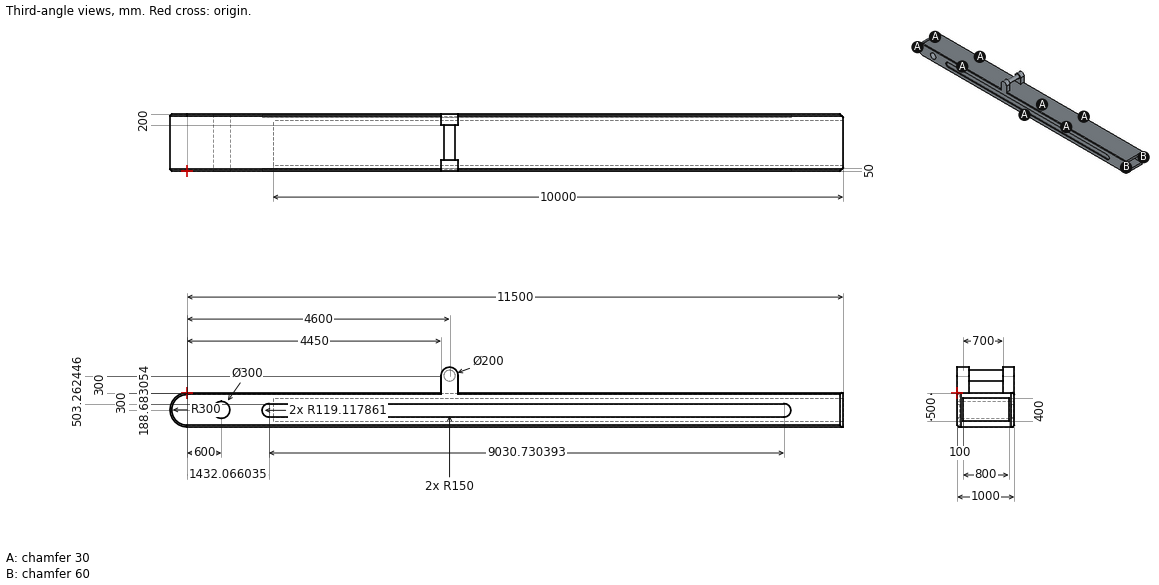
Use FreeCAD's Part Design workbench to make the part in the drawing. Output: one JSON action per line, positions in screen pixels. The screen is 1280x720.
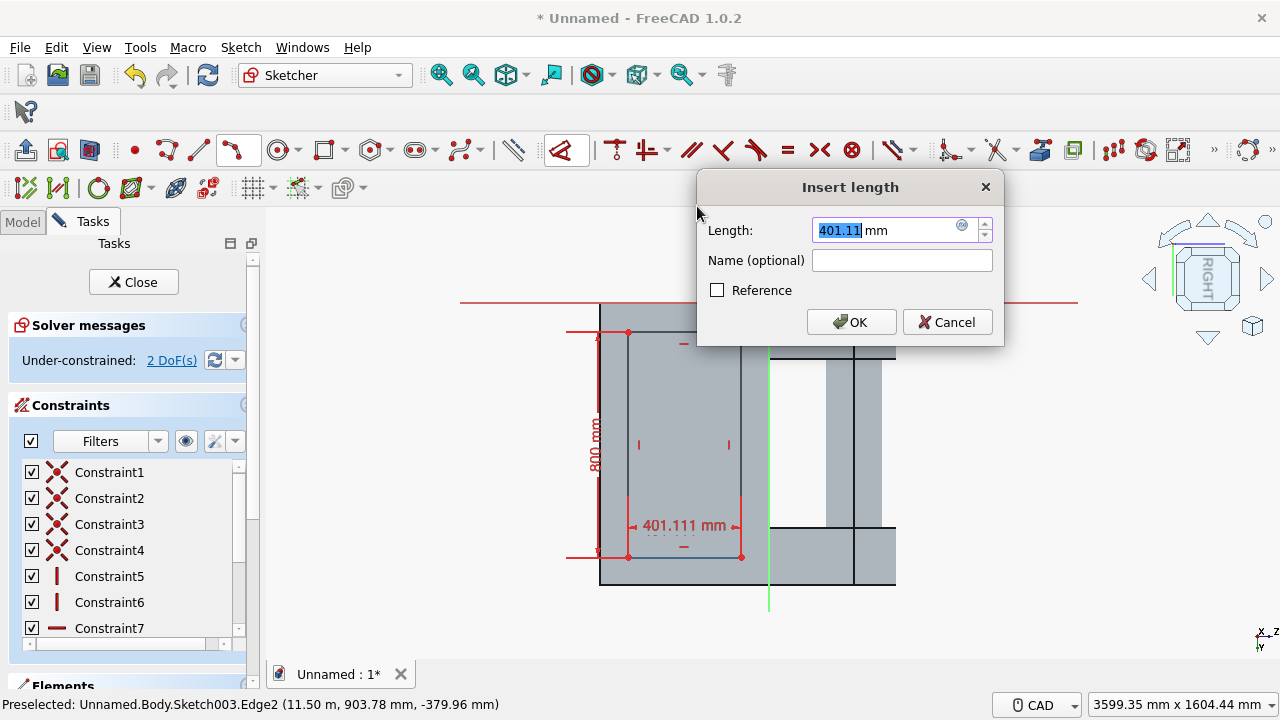
{"action": "type", "text": "400"}
{"action": "key", "text": "Return"}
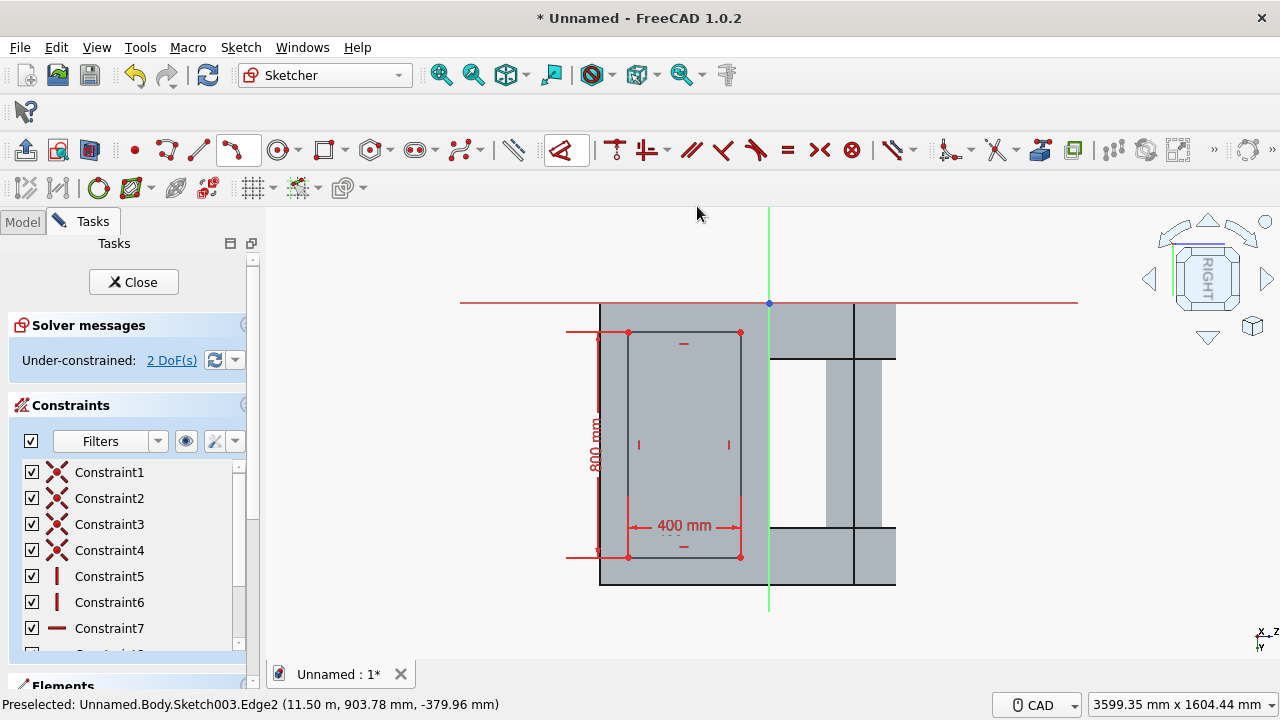
{"action": "left_click", "coordinate": [628, 332]}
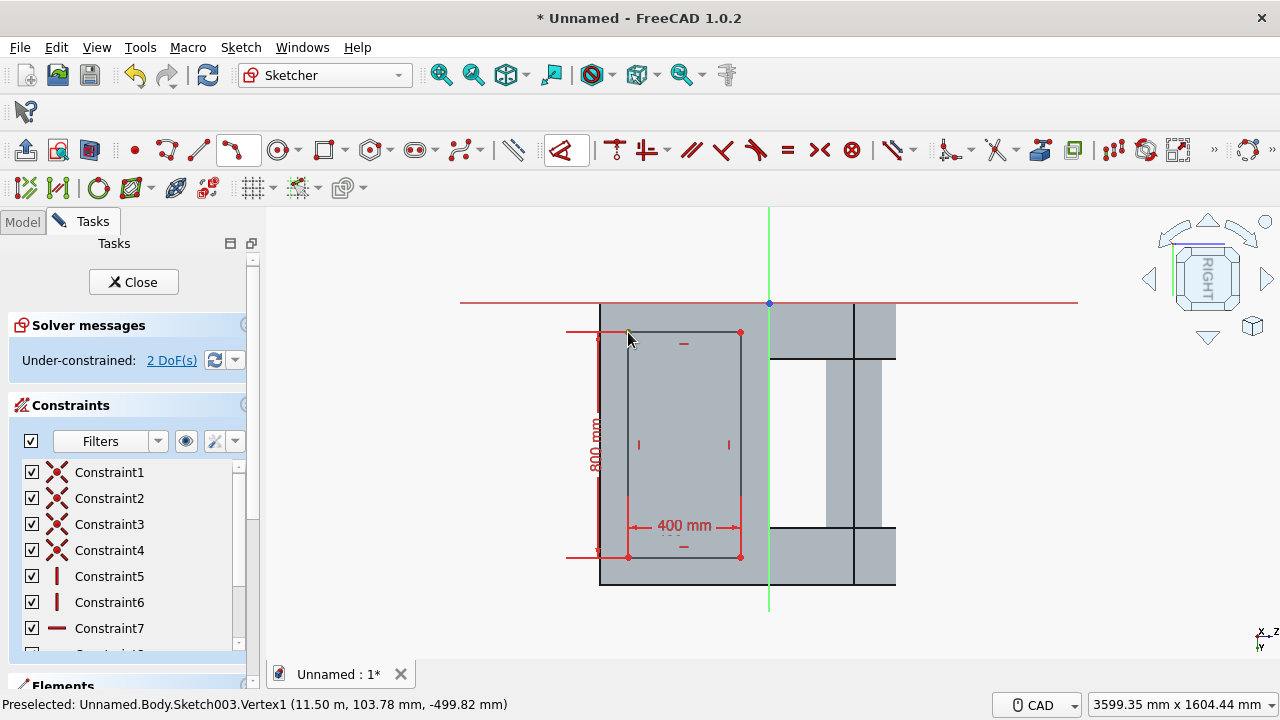
{"action": "left_click", "coordinate": [584, 150]}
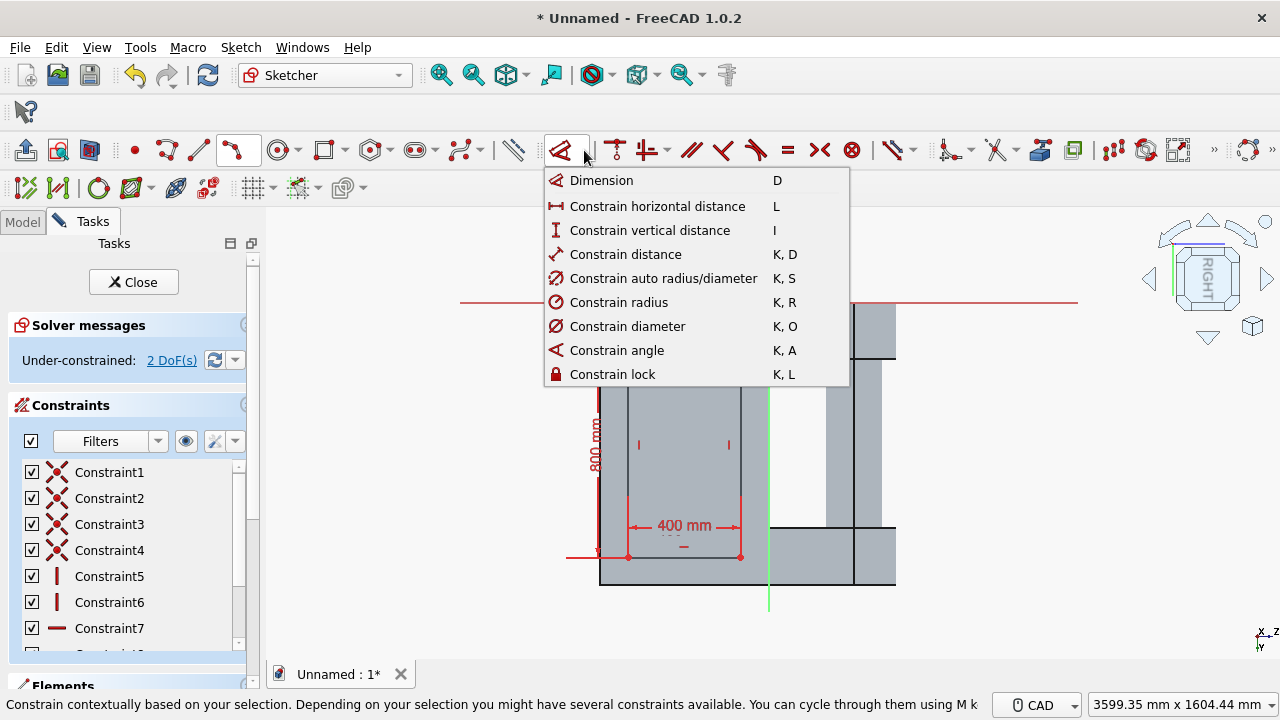
{"action": "left_click", "coordinate": [697, 206]}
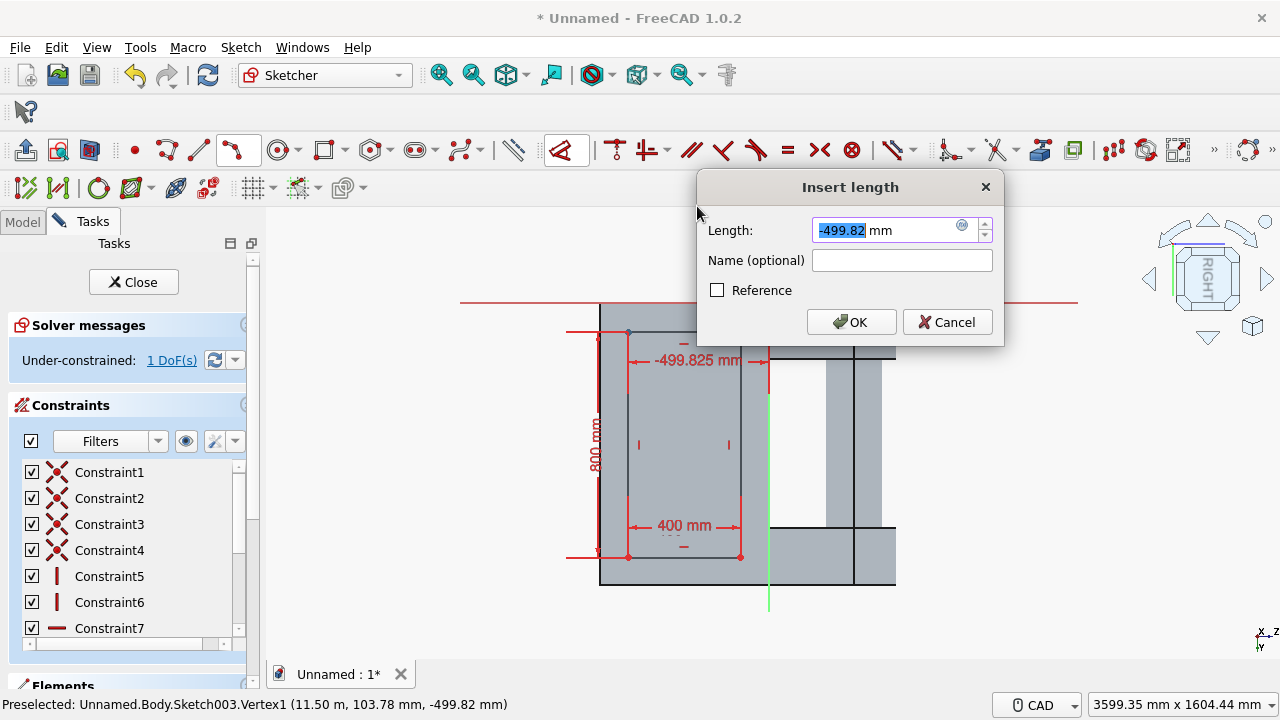
{"action": "type", "text": "-500"}
{"action": "key", "text": "Return"}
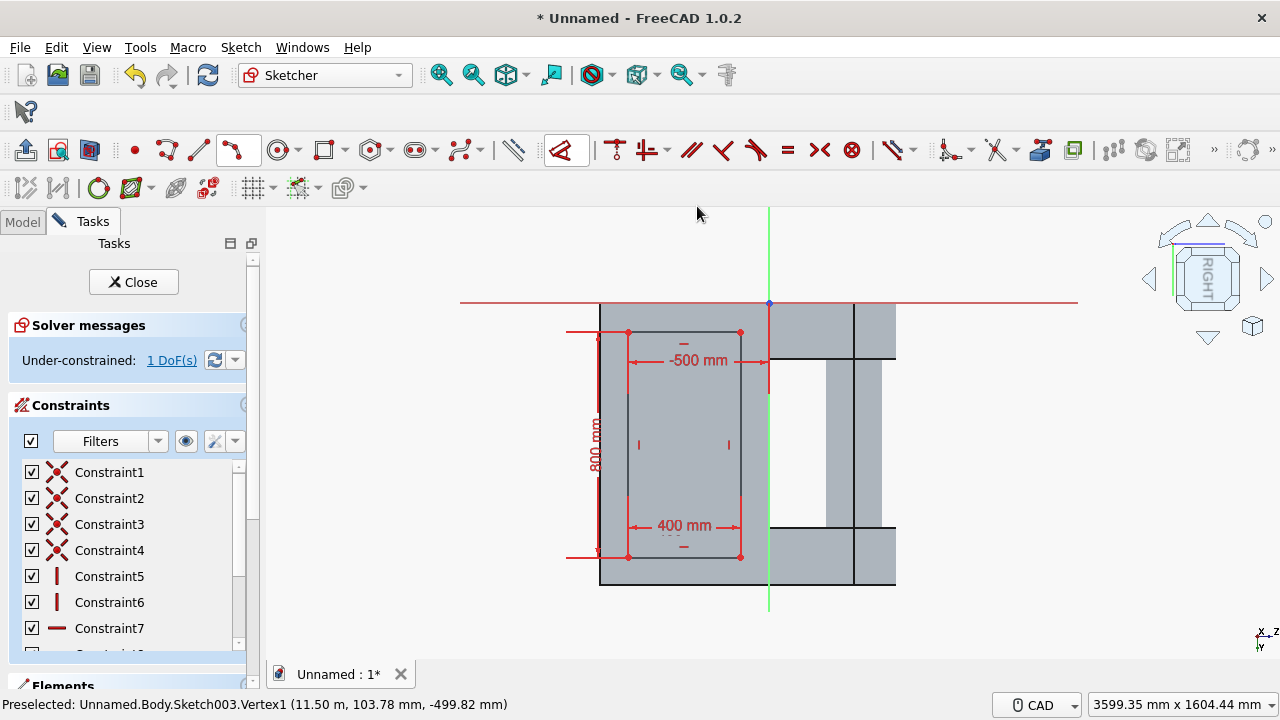
{"action": "scroll", "coordinate": [628, 332], "scroll_direction": "up", "scroll_amount": 2}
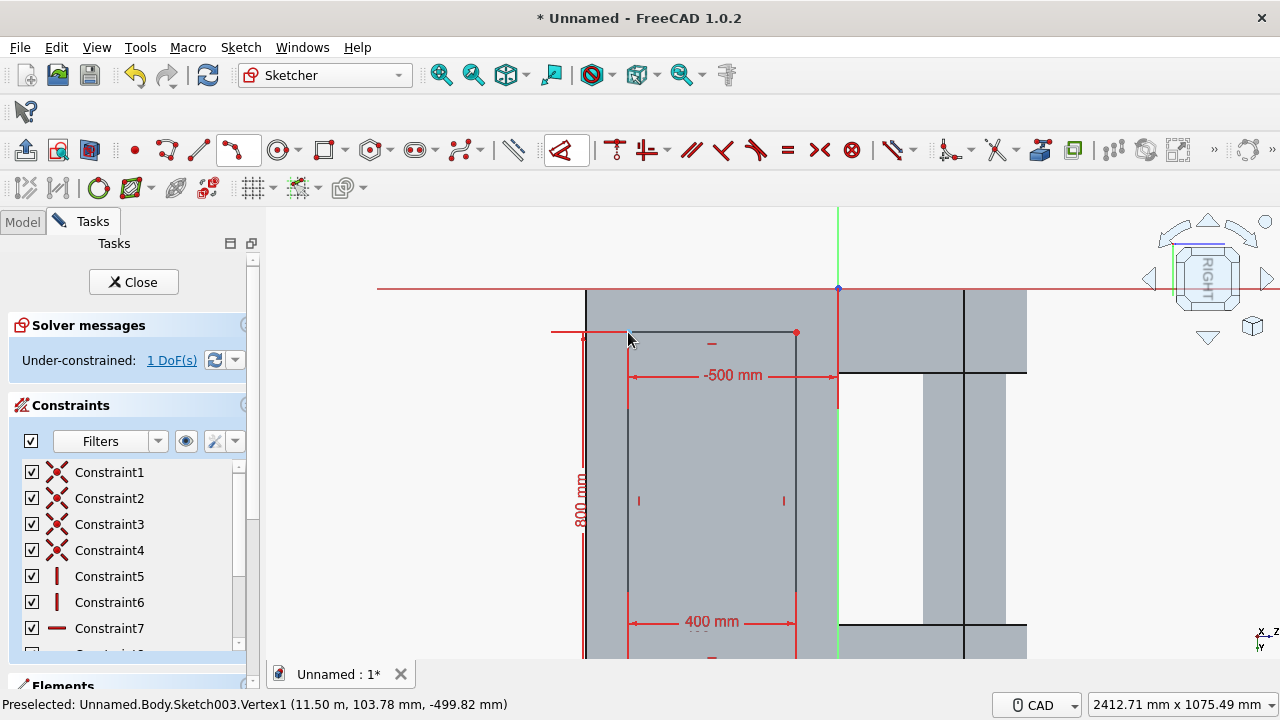
{"action": "left_click", "coordinate": [628, 332]}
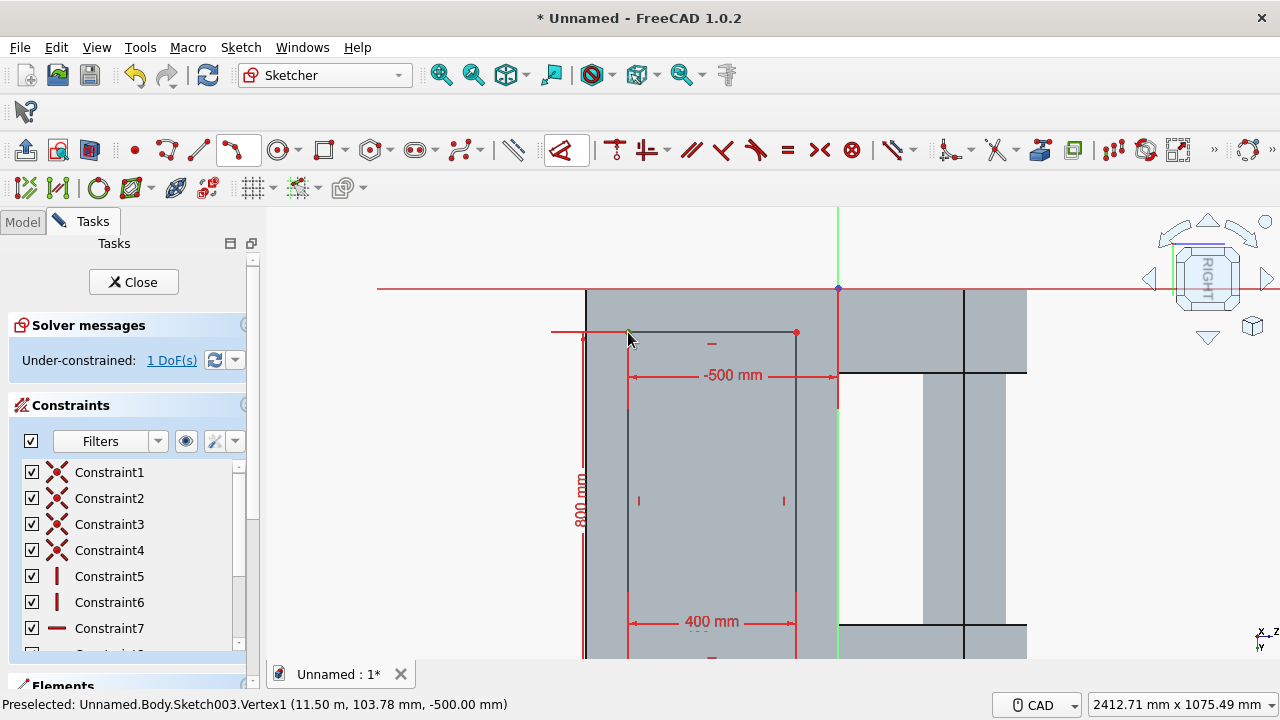
{"action": "key", "text": "i"}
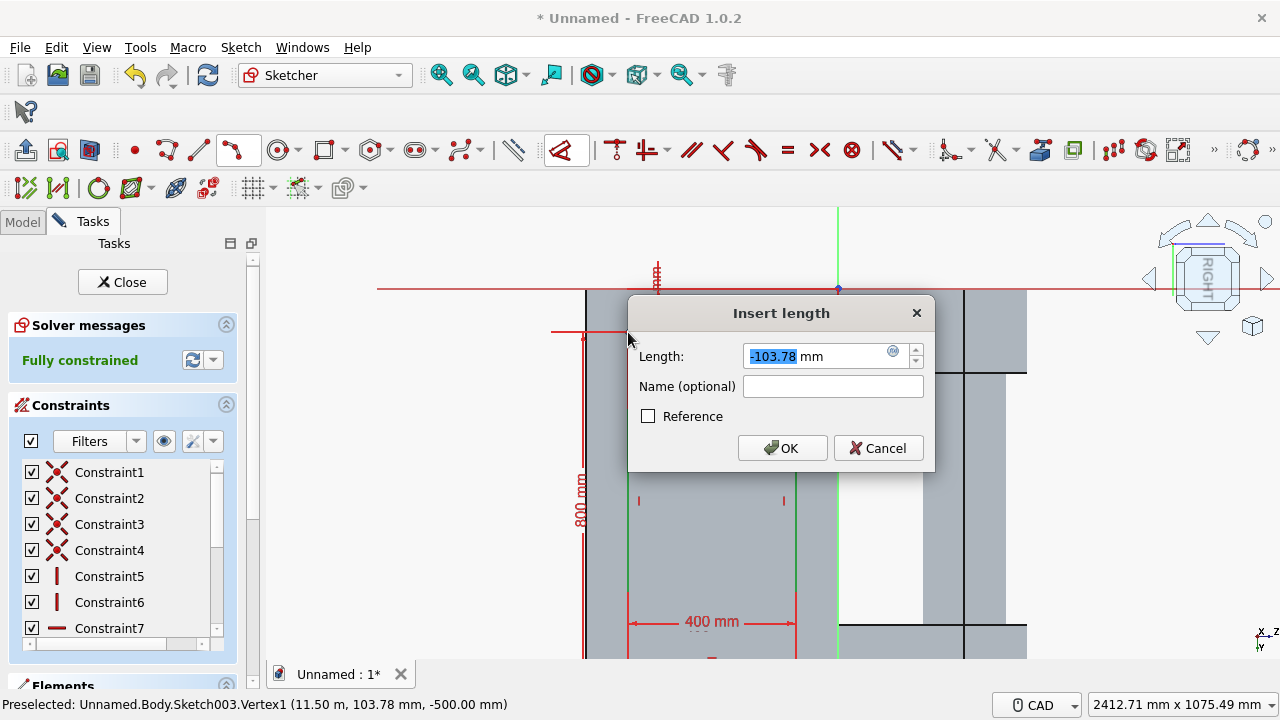
{"action": "type", "text": "-100"}
{"action": "key", "text": "Return"}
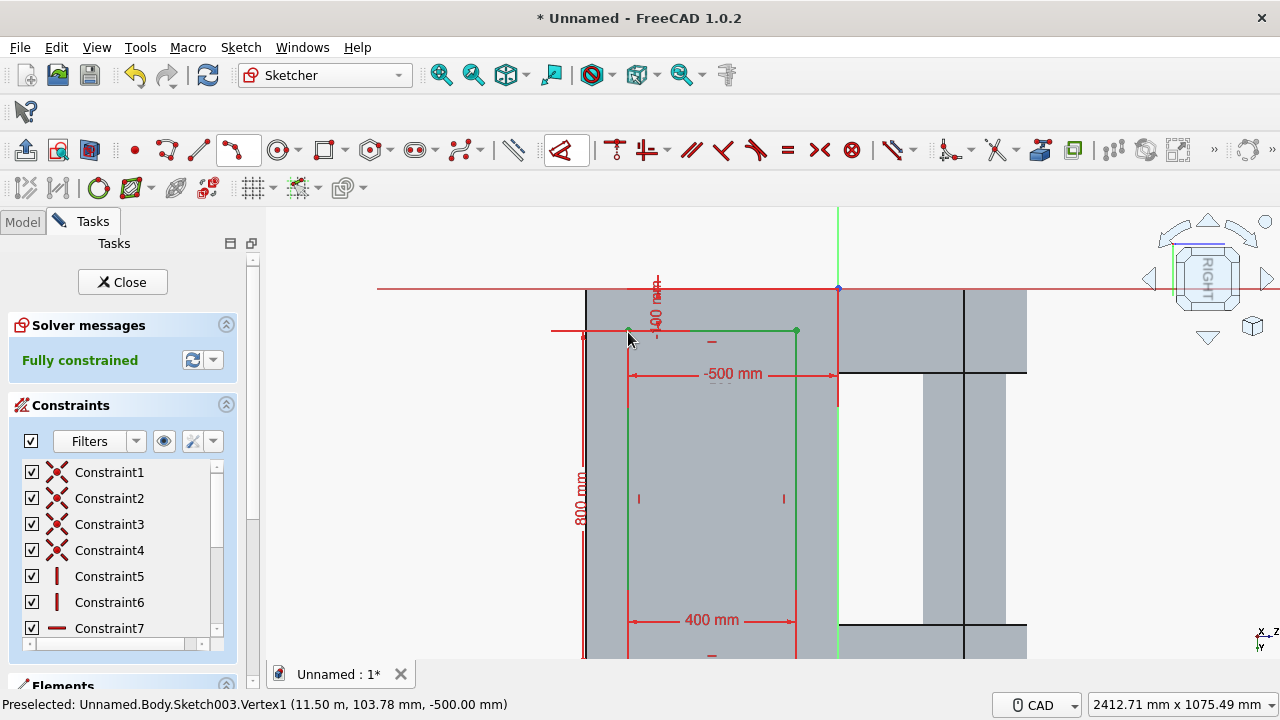
{"action": "left_click", "coordinate": [123, 282]}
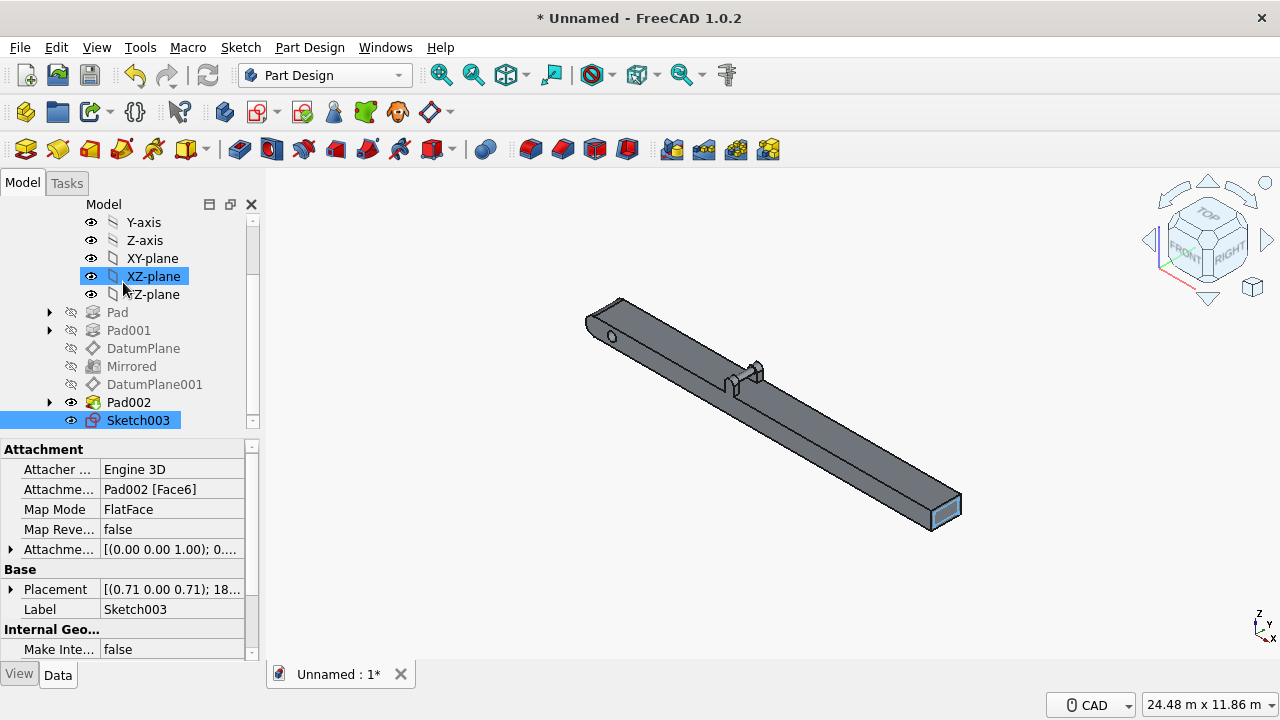
{"action": "left_click", "coordinate": [240, 150]}